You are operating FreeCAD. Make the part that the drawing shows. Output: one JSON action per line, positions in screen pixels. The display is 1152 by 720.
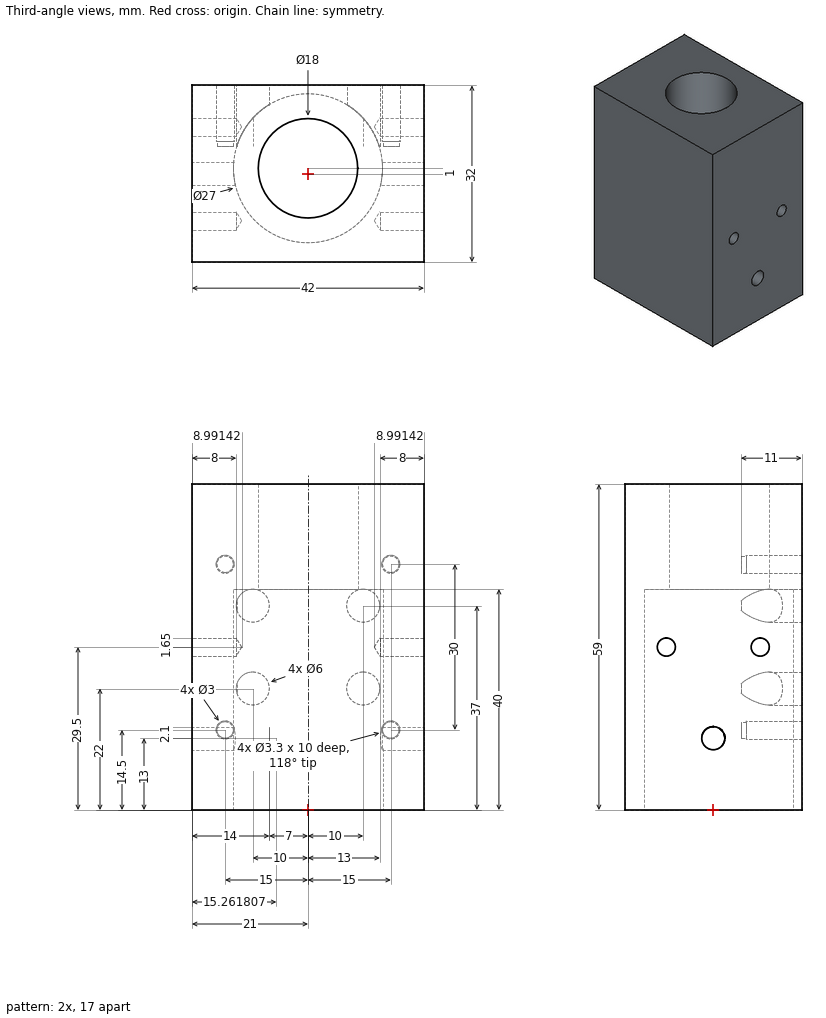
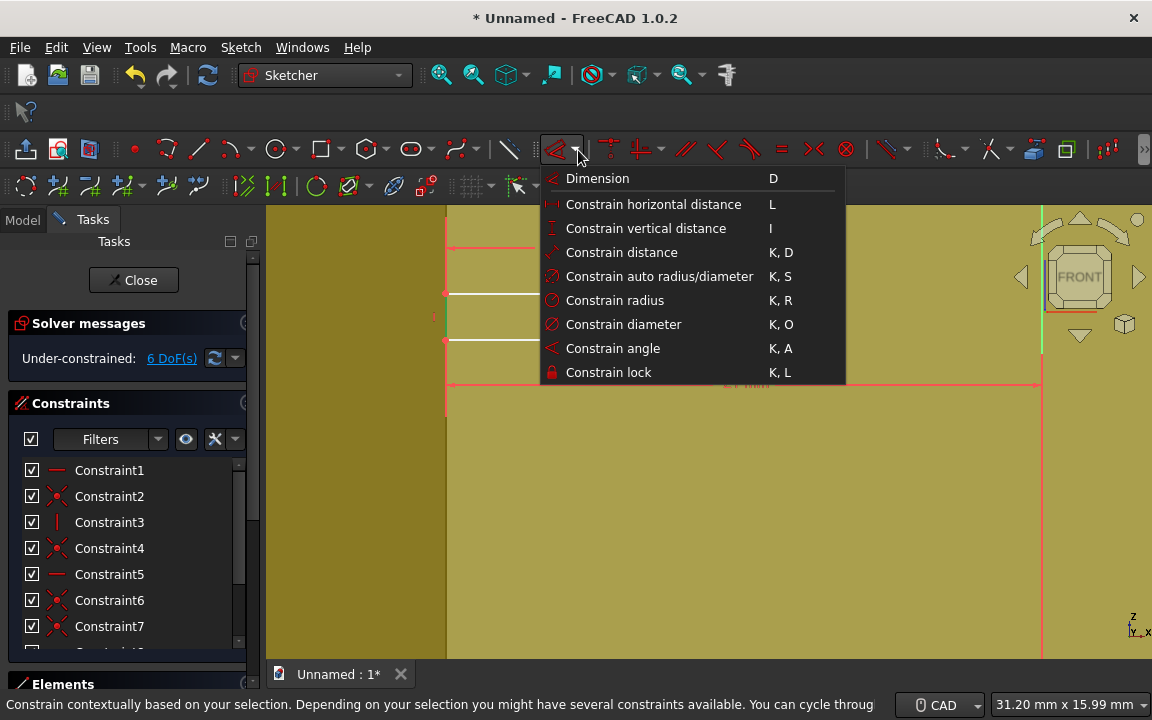
{"action": "left_click", "coordinate": [693, 228]}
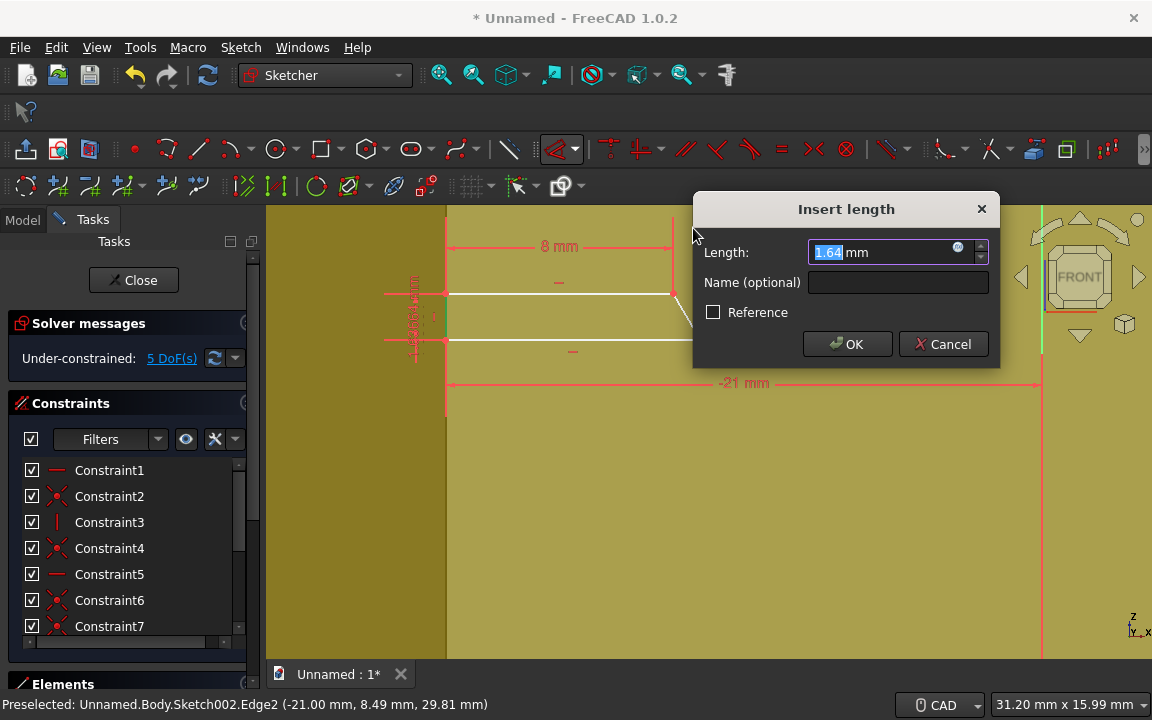
{"action": "type", "text": "1.65"}
{"action": "key", "text": "Return"}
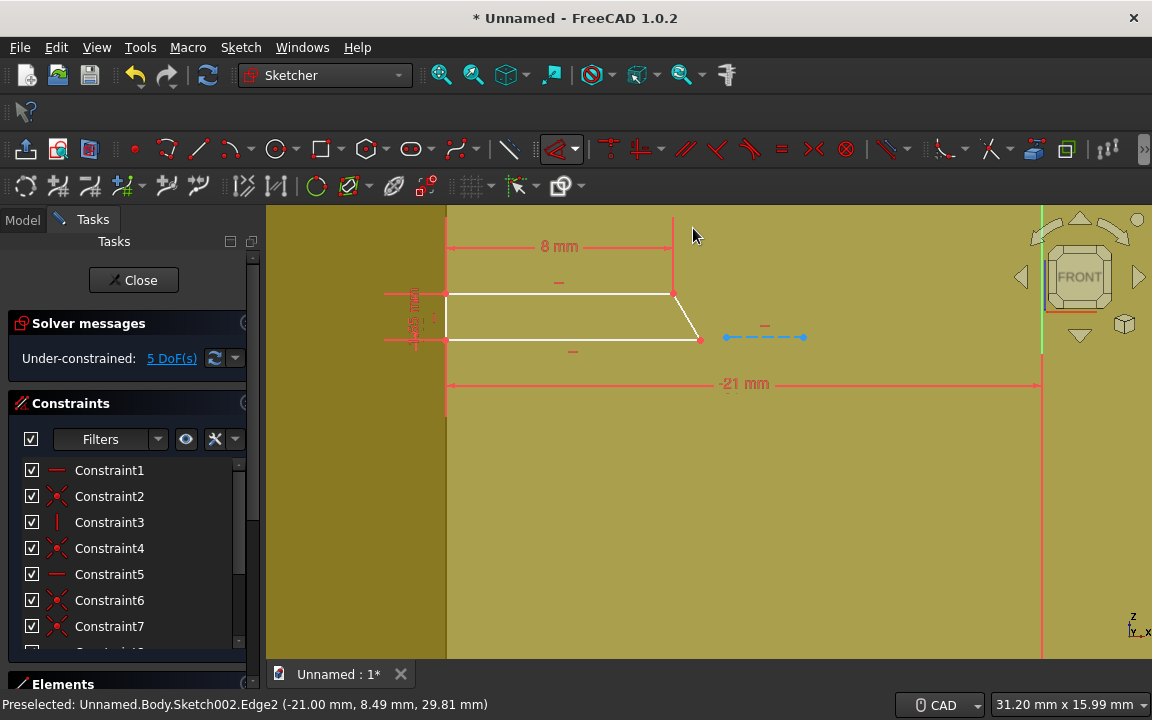
{"action": "left_click", "coordinate": [701, 340]}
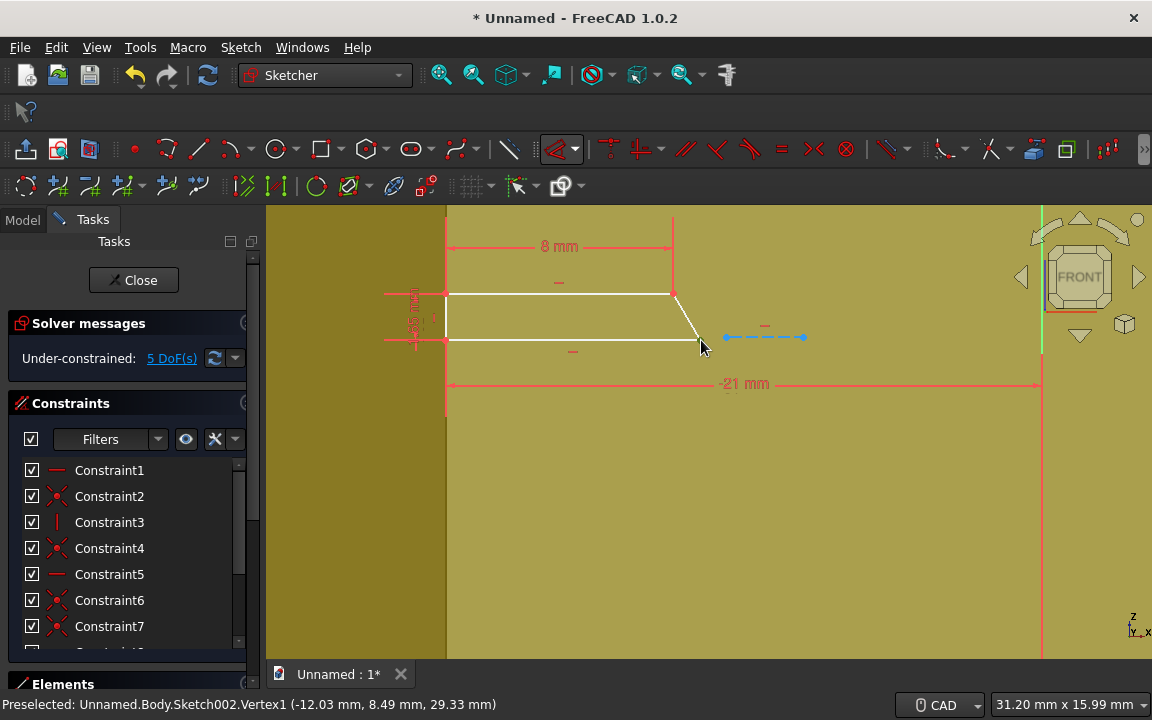
{"action": "key", "text": "i"}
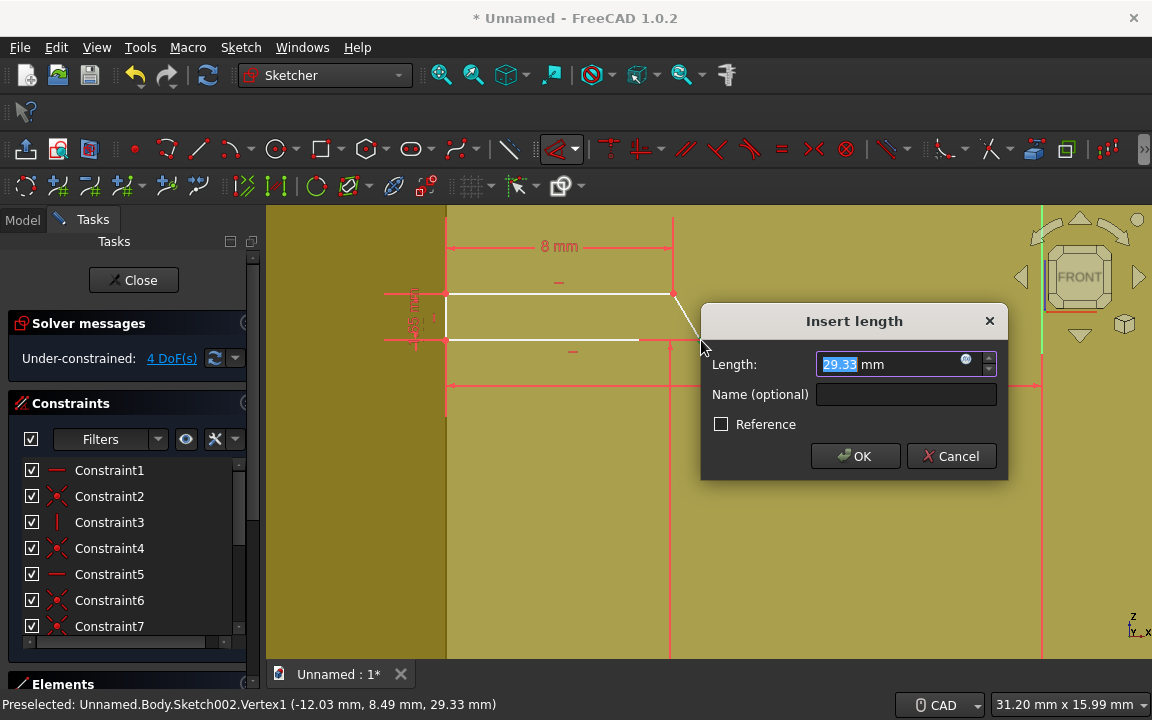
{"action": "type", "text": "29.5"}
{"action": "key", "text": "Return"}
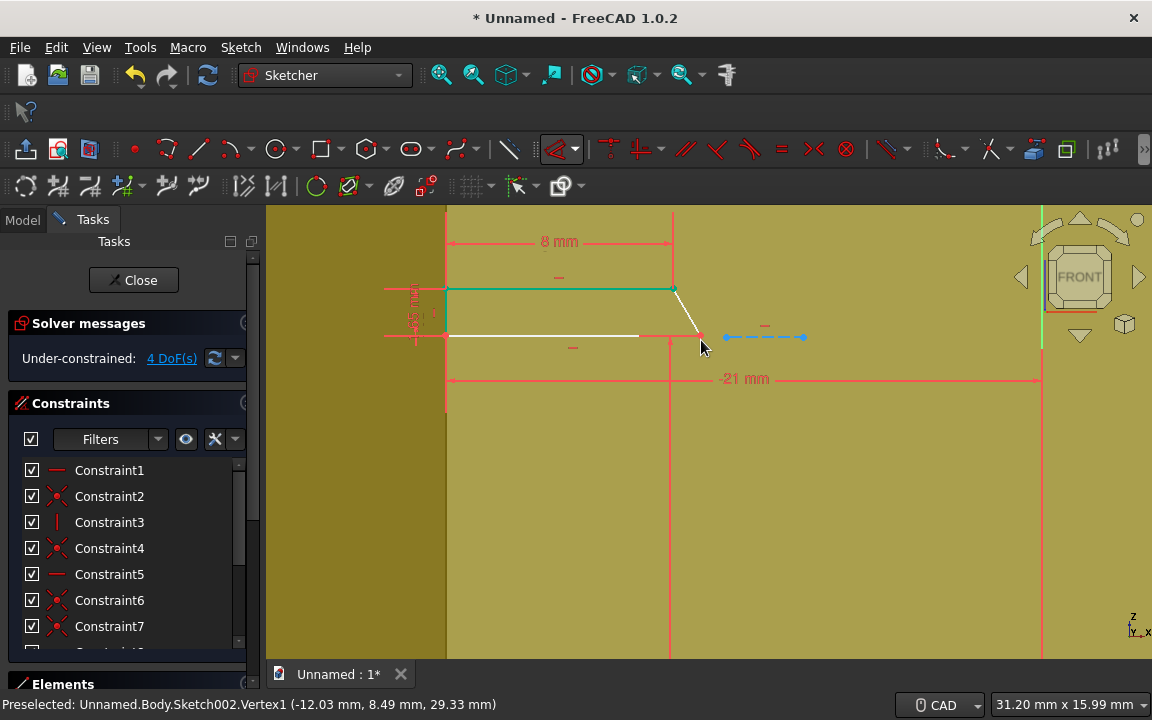
{"action": "left_click", "coordinate": [726, 337]}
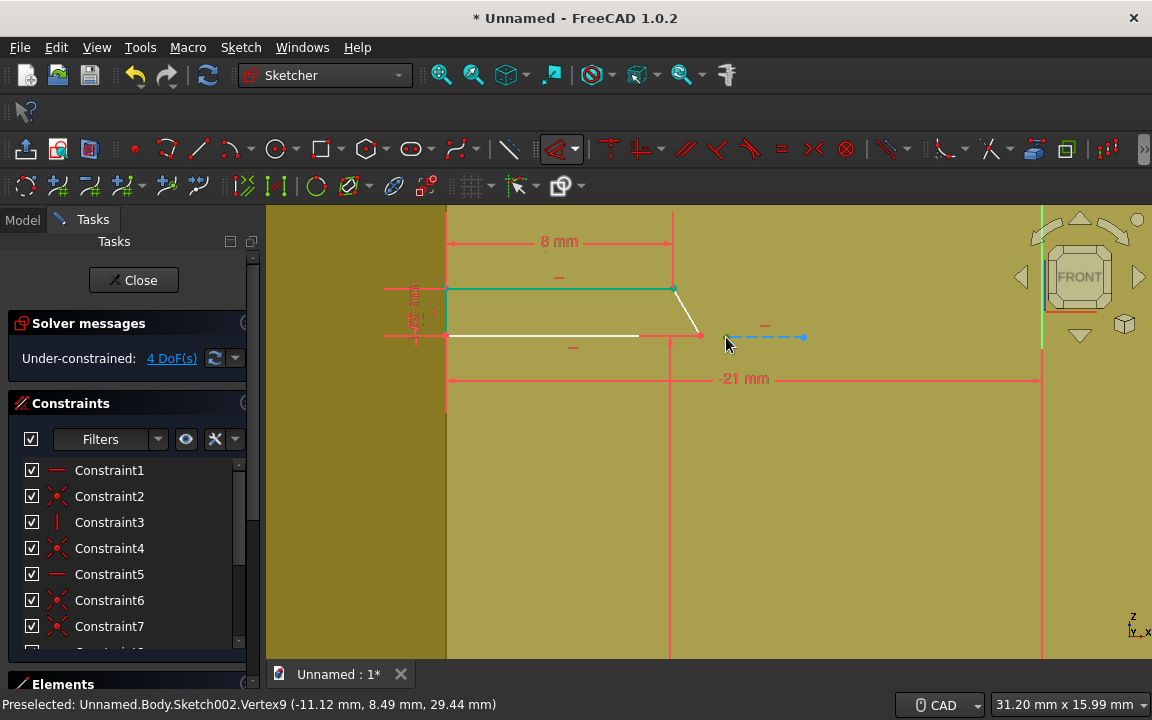
{"action": "left_click", "coordinate": [578, 150]}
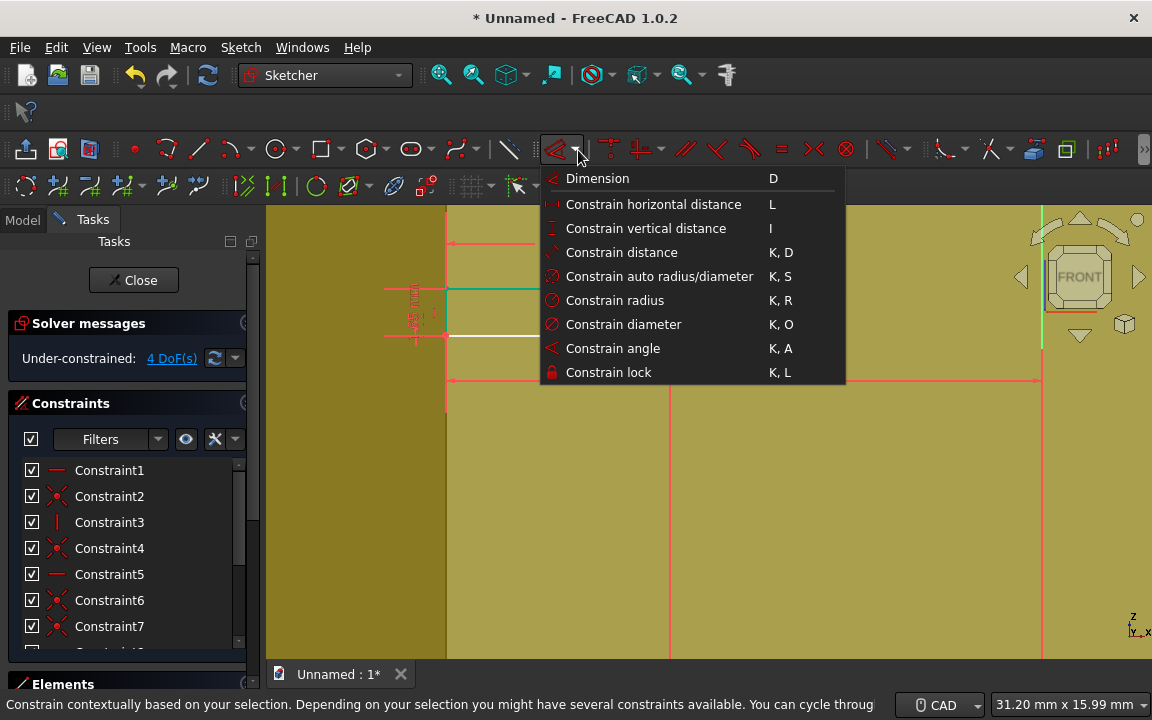
{"action": "left_click", "coordinate": [693, 228]}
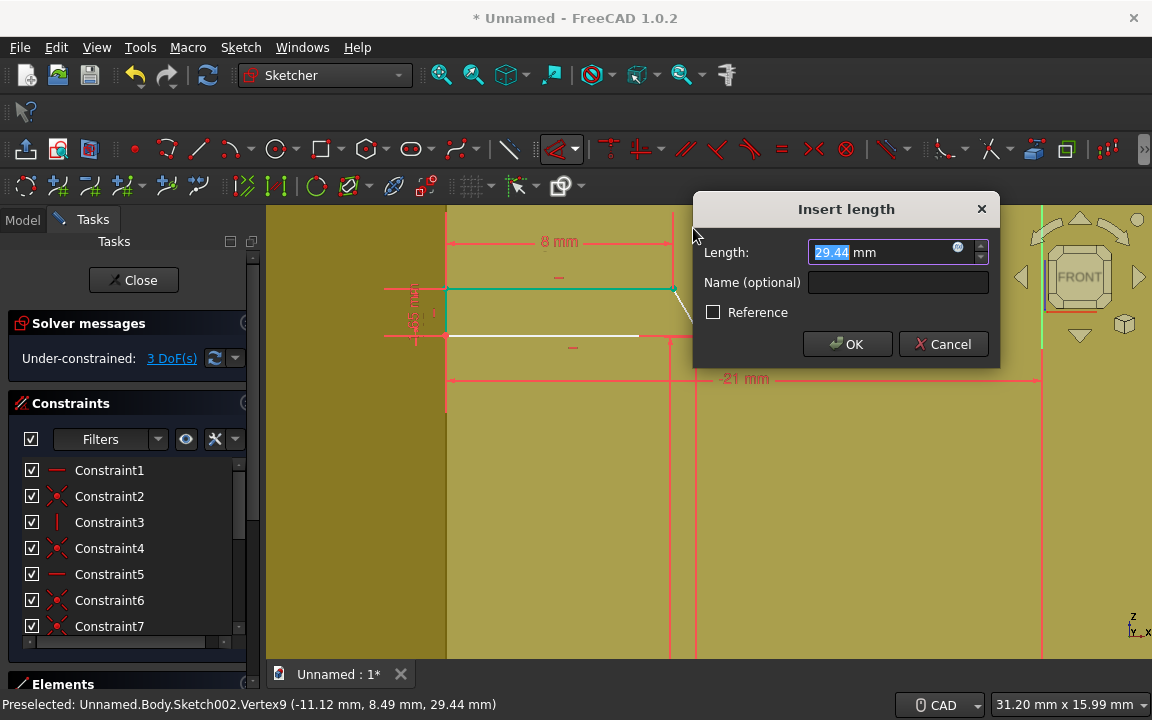
{"action": "type", "text": "29.5"}
{"action": "key", "text": "Return"}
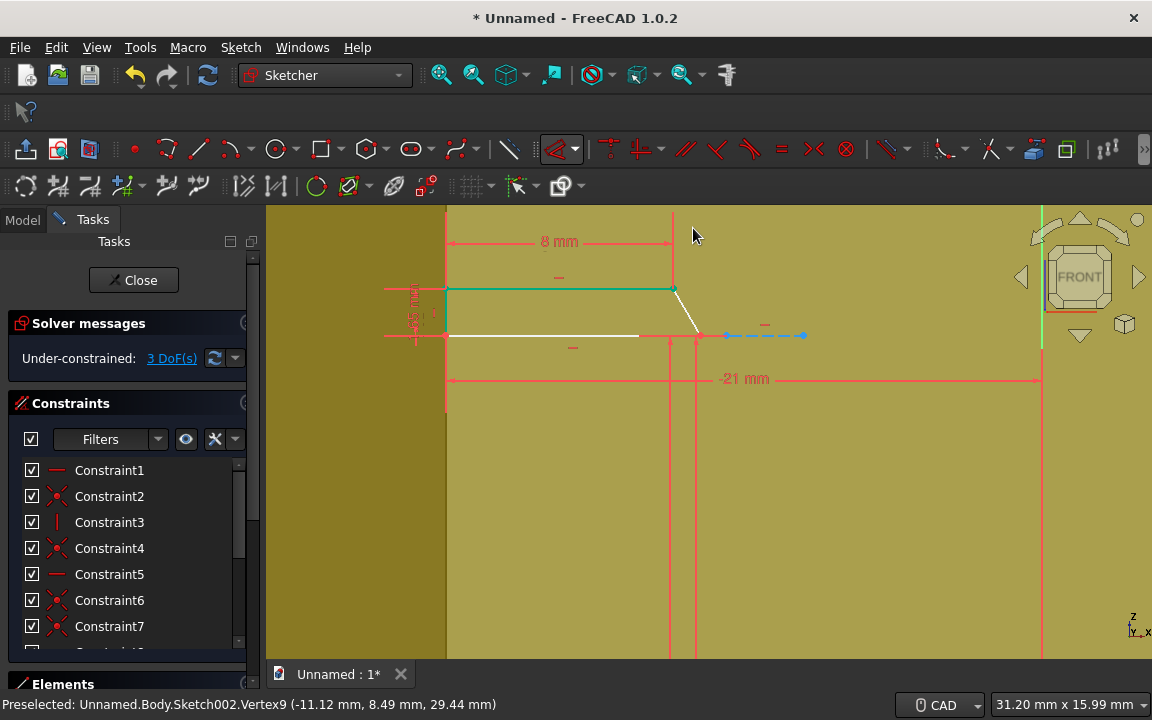
{"action": "left_click", "coordinate": [624, 336]}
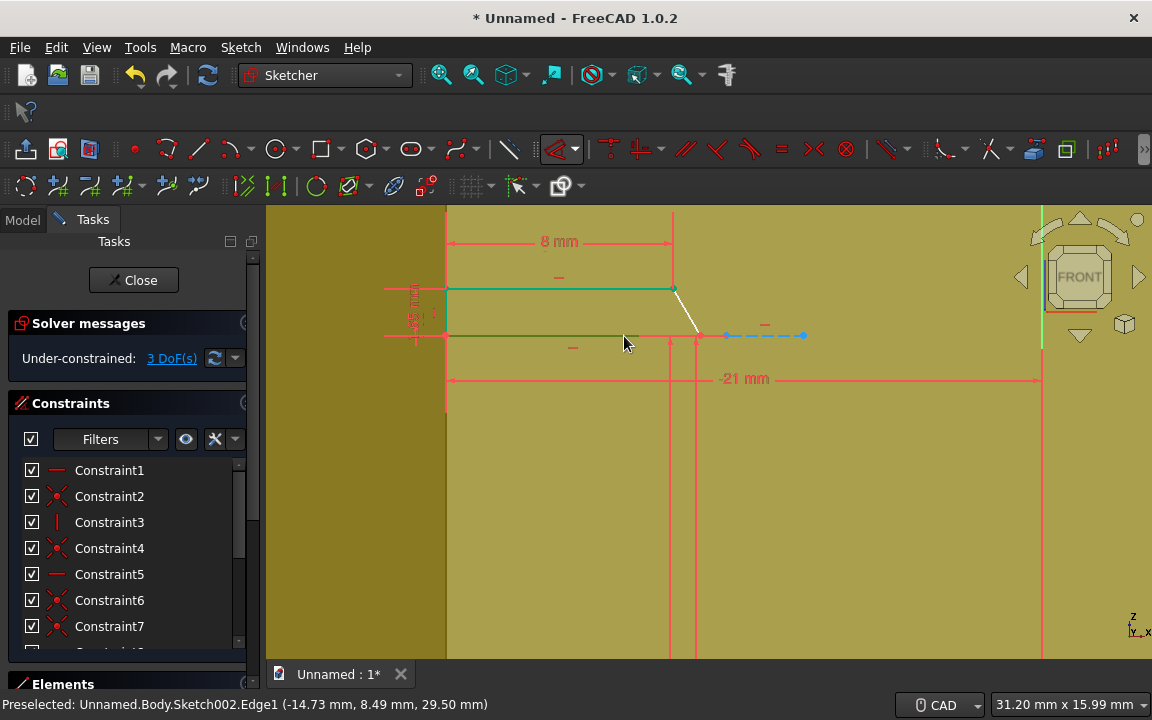
{"action": "key", "text": "l"}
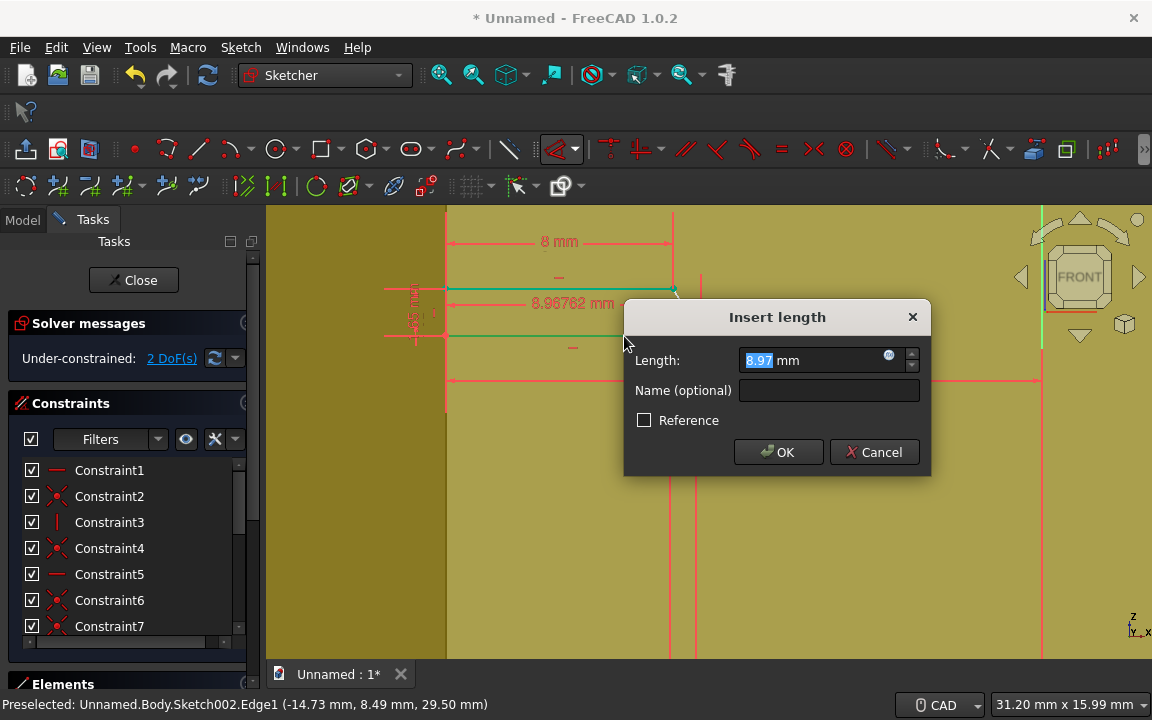
{"action": "type", "text": "8.99142"}
{"action": "key", "text": "Return"}